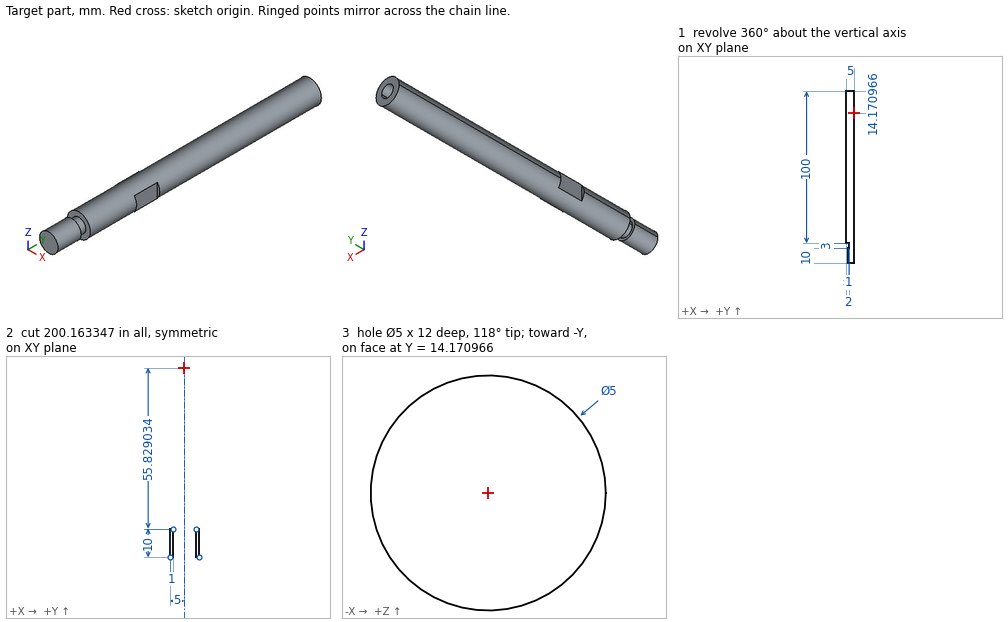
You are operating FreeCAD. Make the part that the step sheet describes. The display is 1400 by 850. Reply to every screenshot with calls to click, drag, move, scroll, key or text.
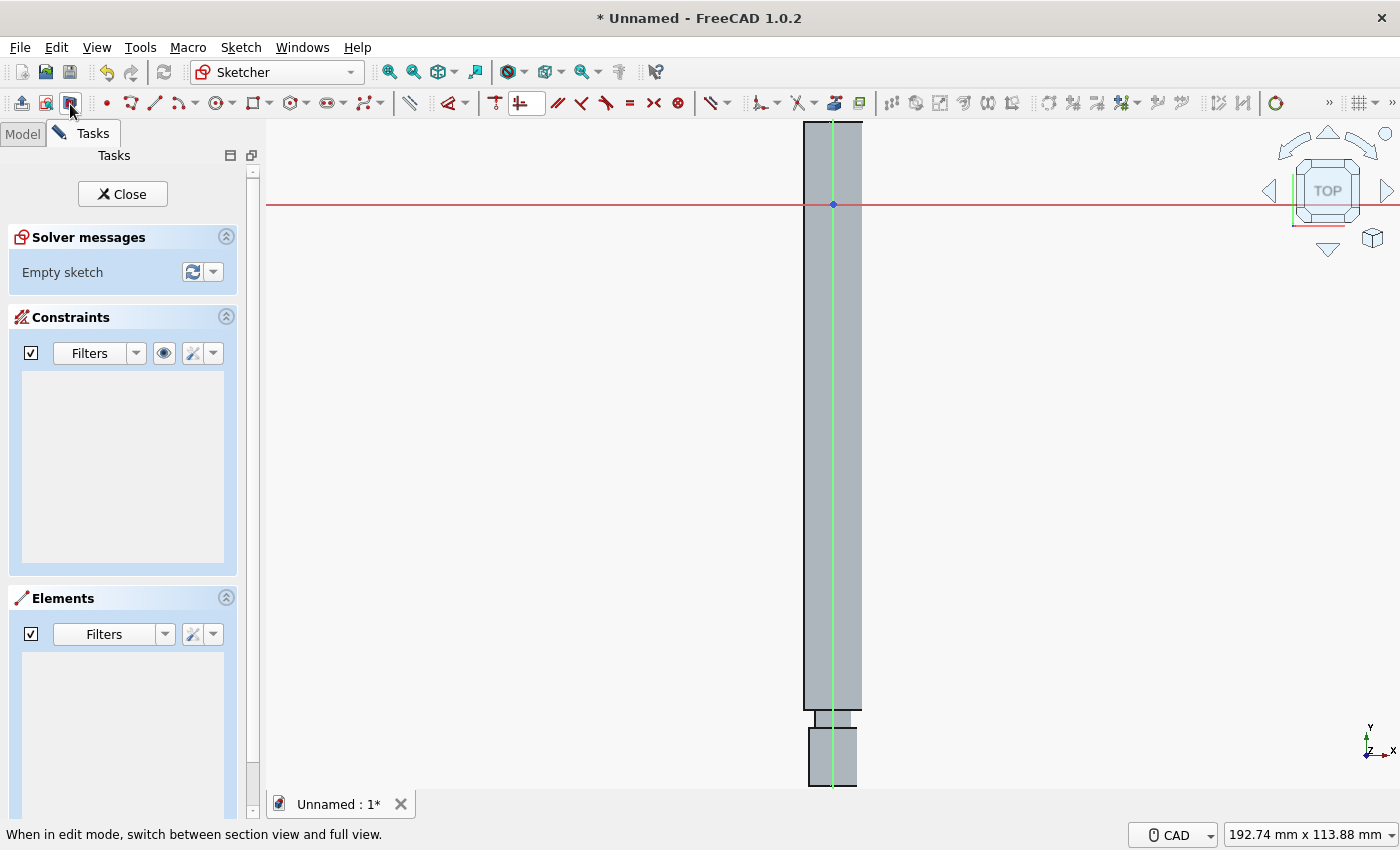
scroll(844, 580, up, 10)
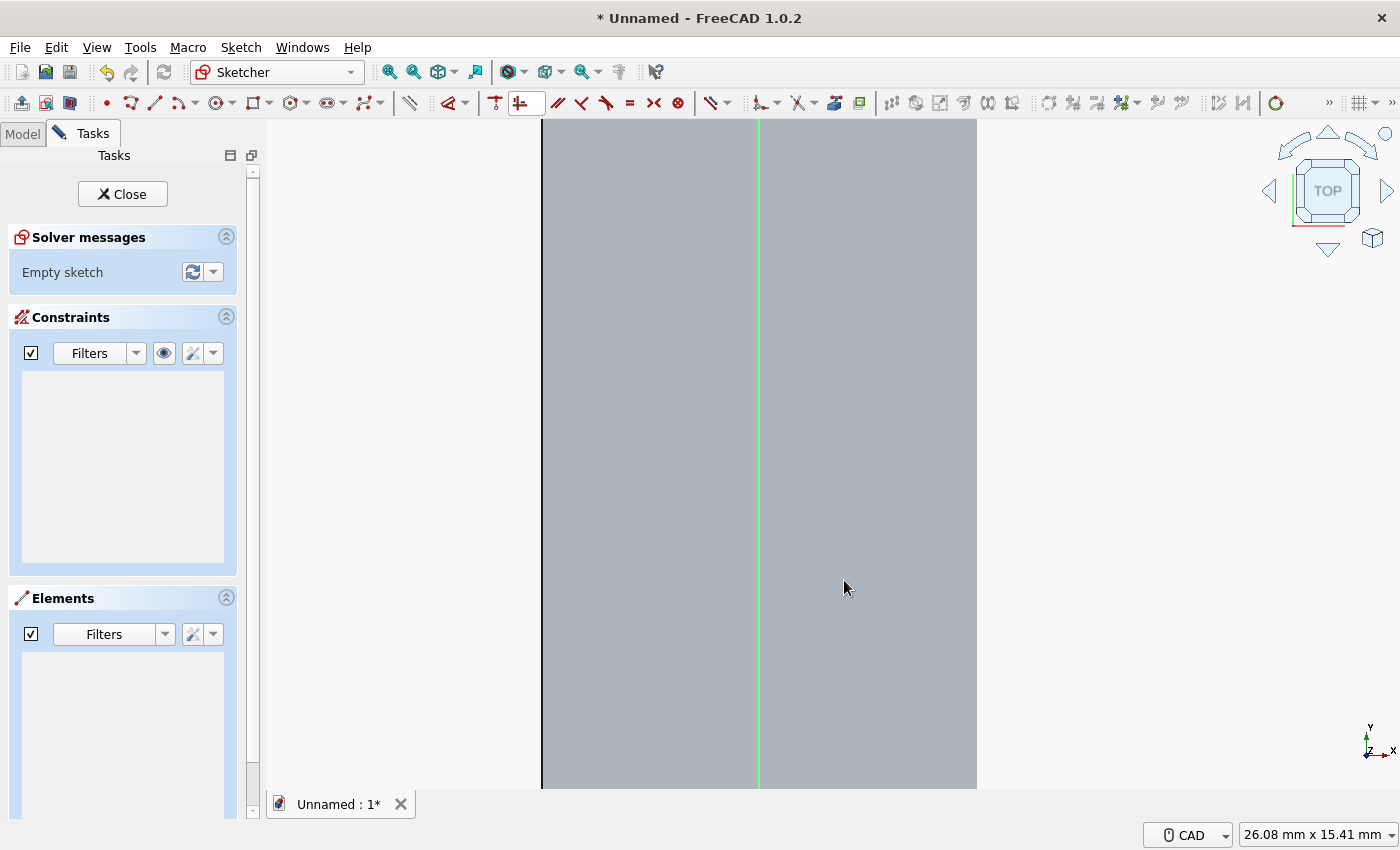
click(254, 104)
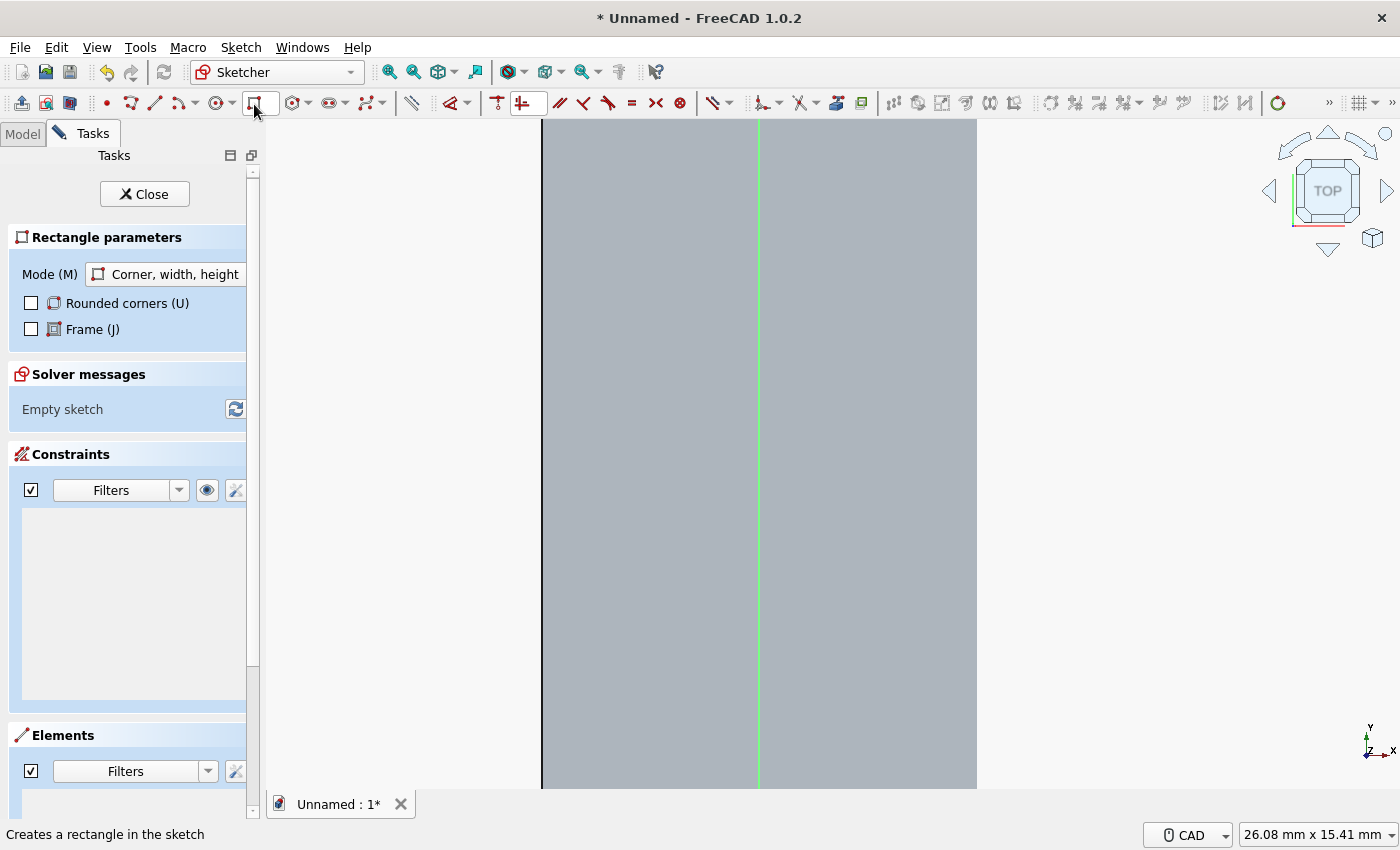
click(542, 231)
click(586, 666)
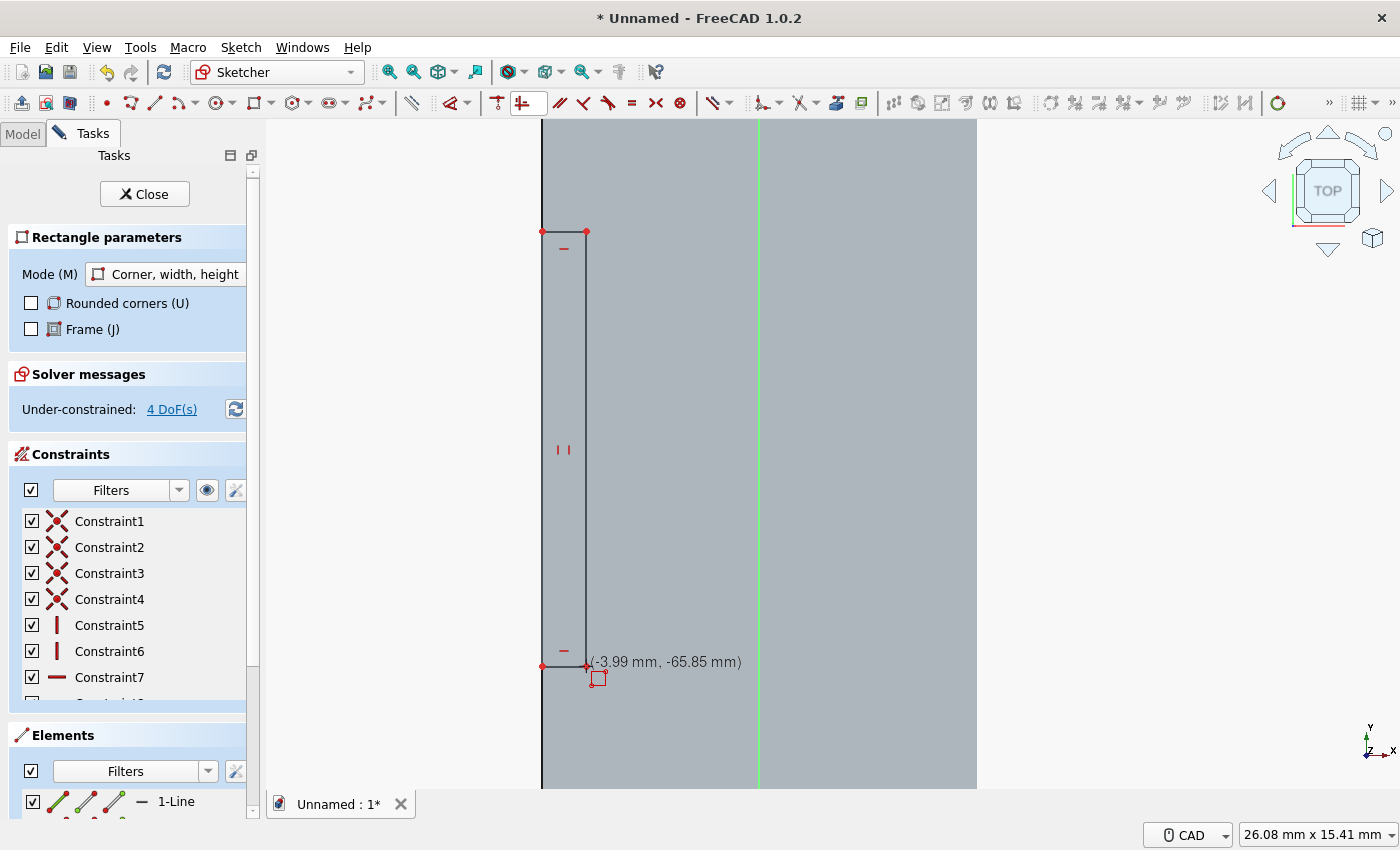
click(933, 231)
click(977, 666)
key(Escape)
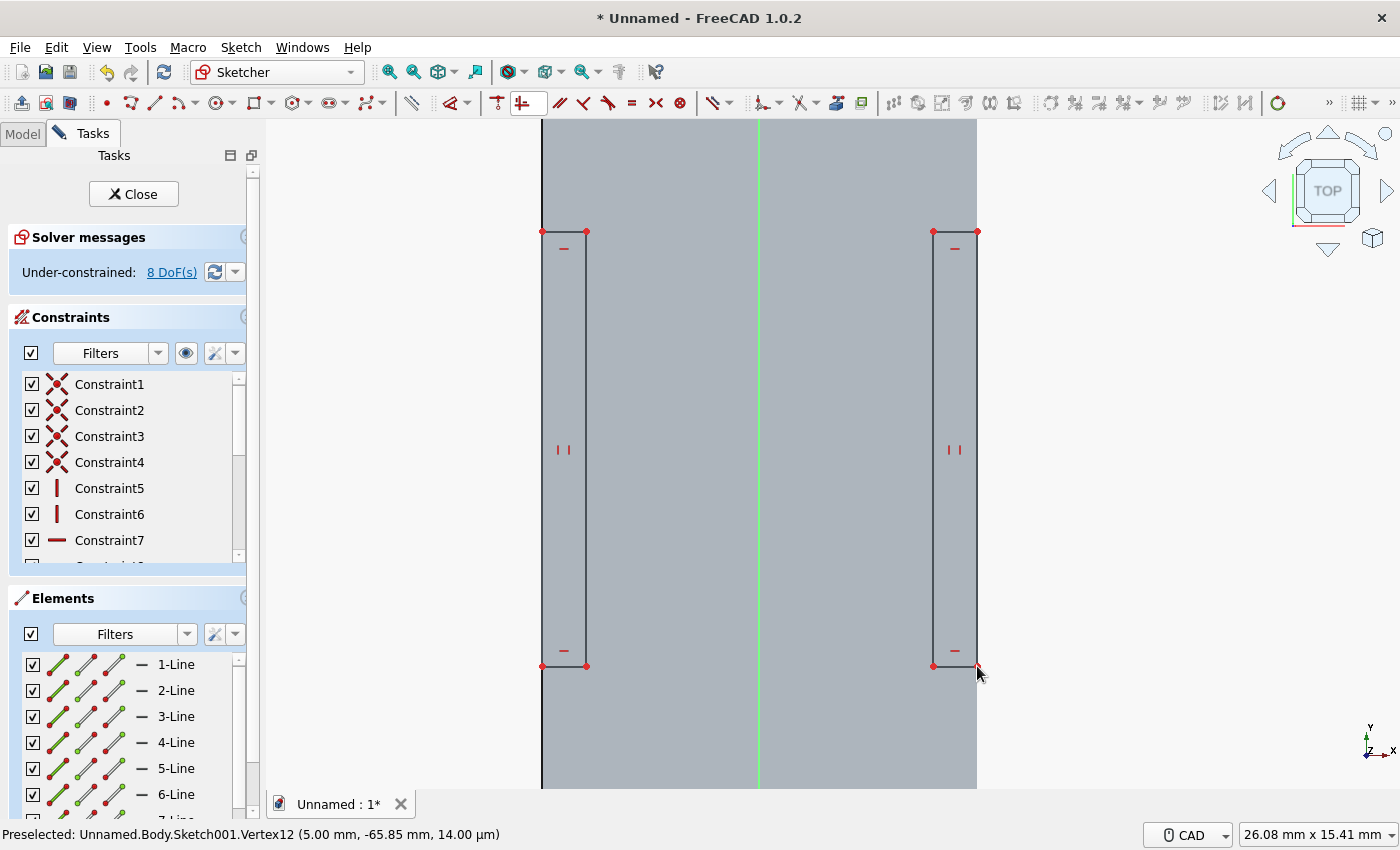
click(586, 232)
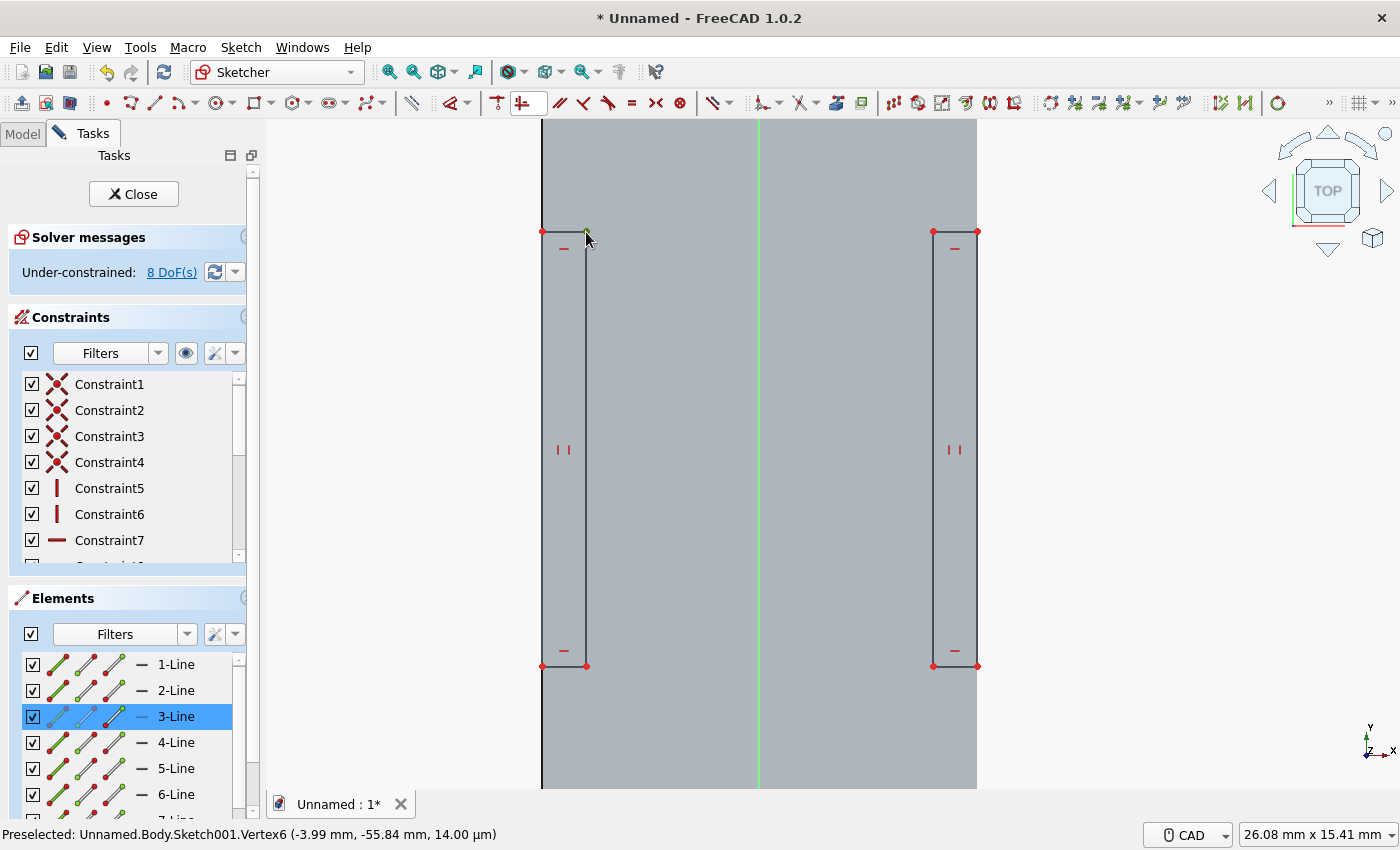
click(933, 232)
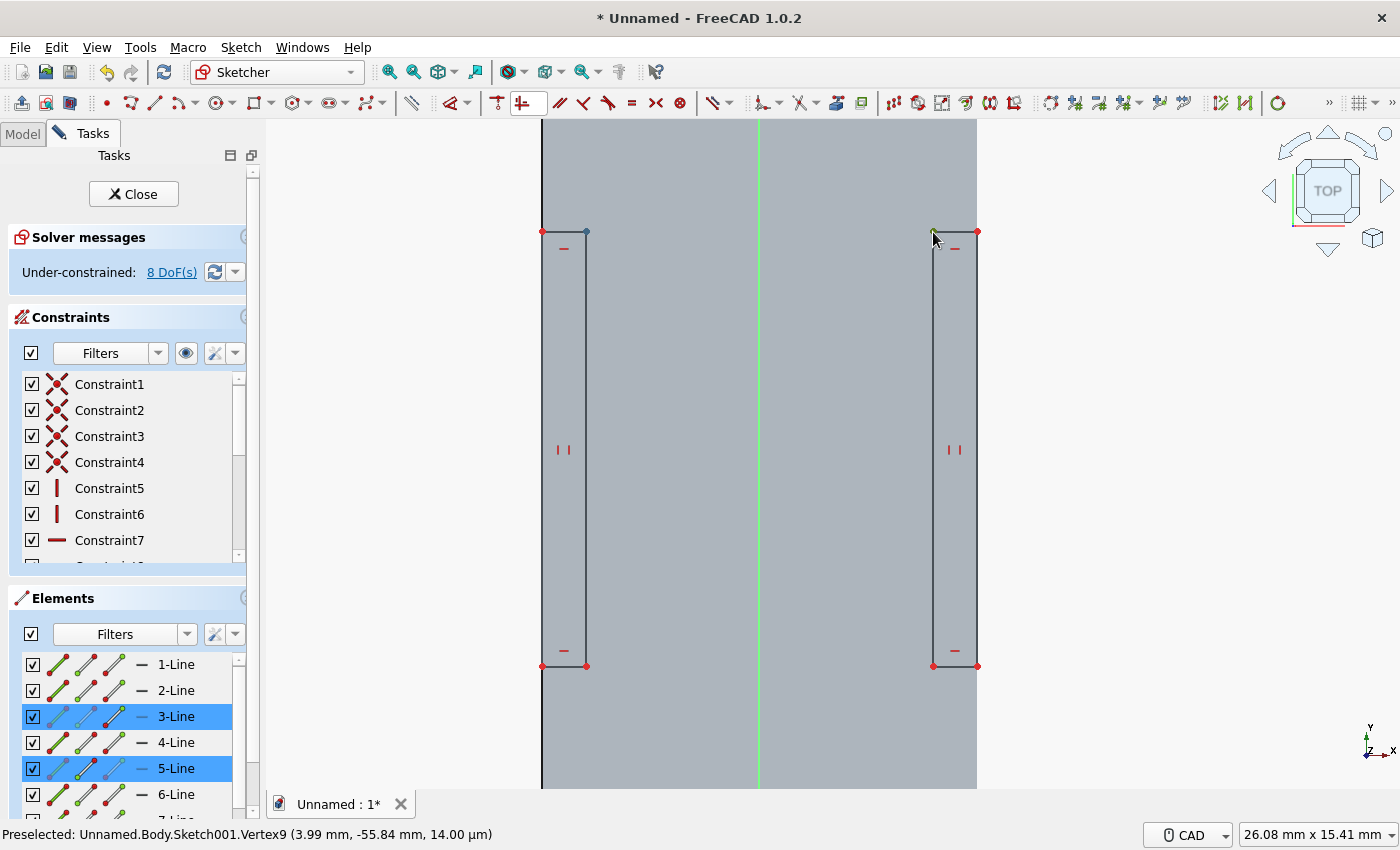
click(759, 717)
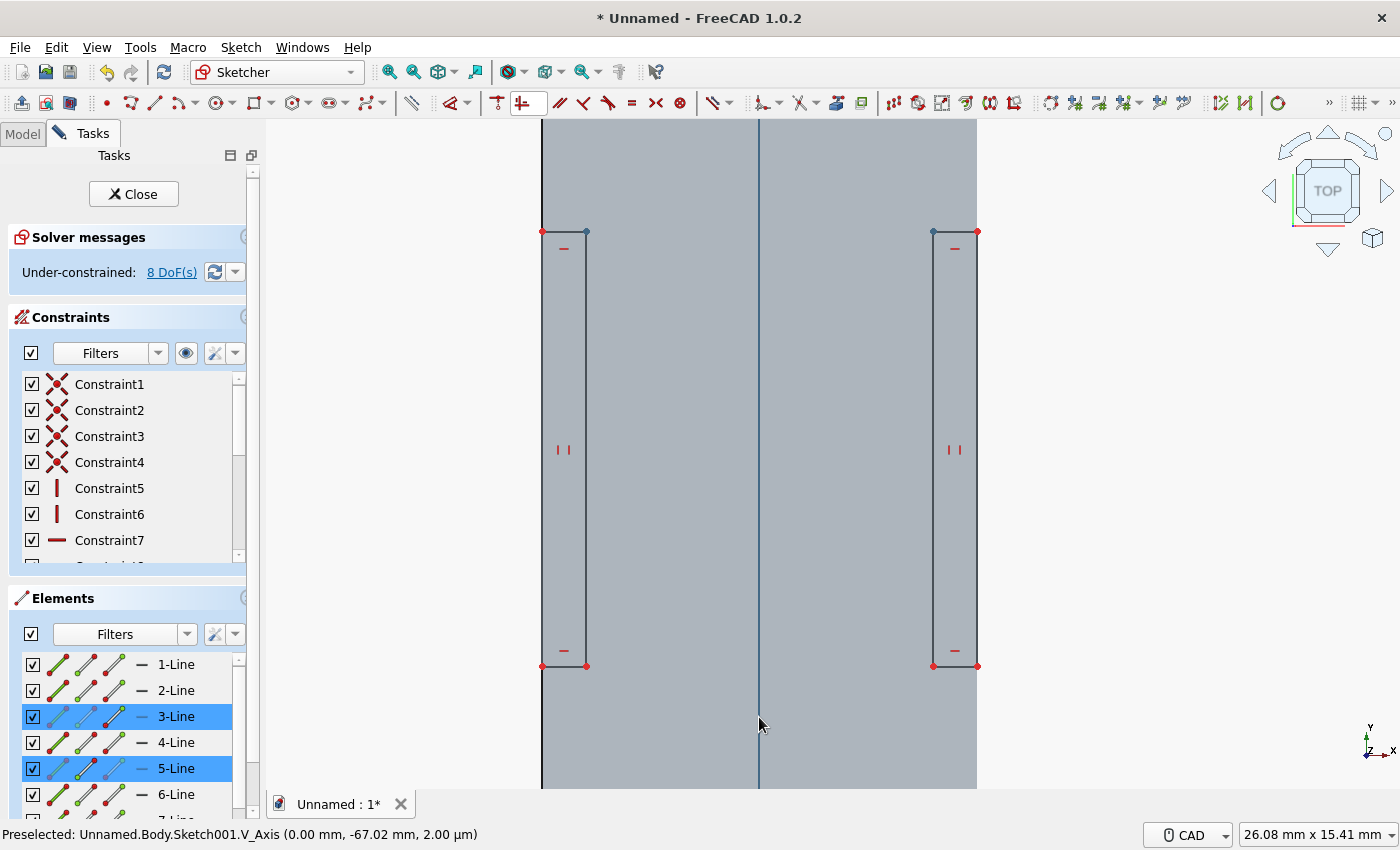
click(656, 104)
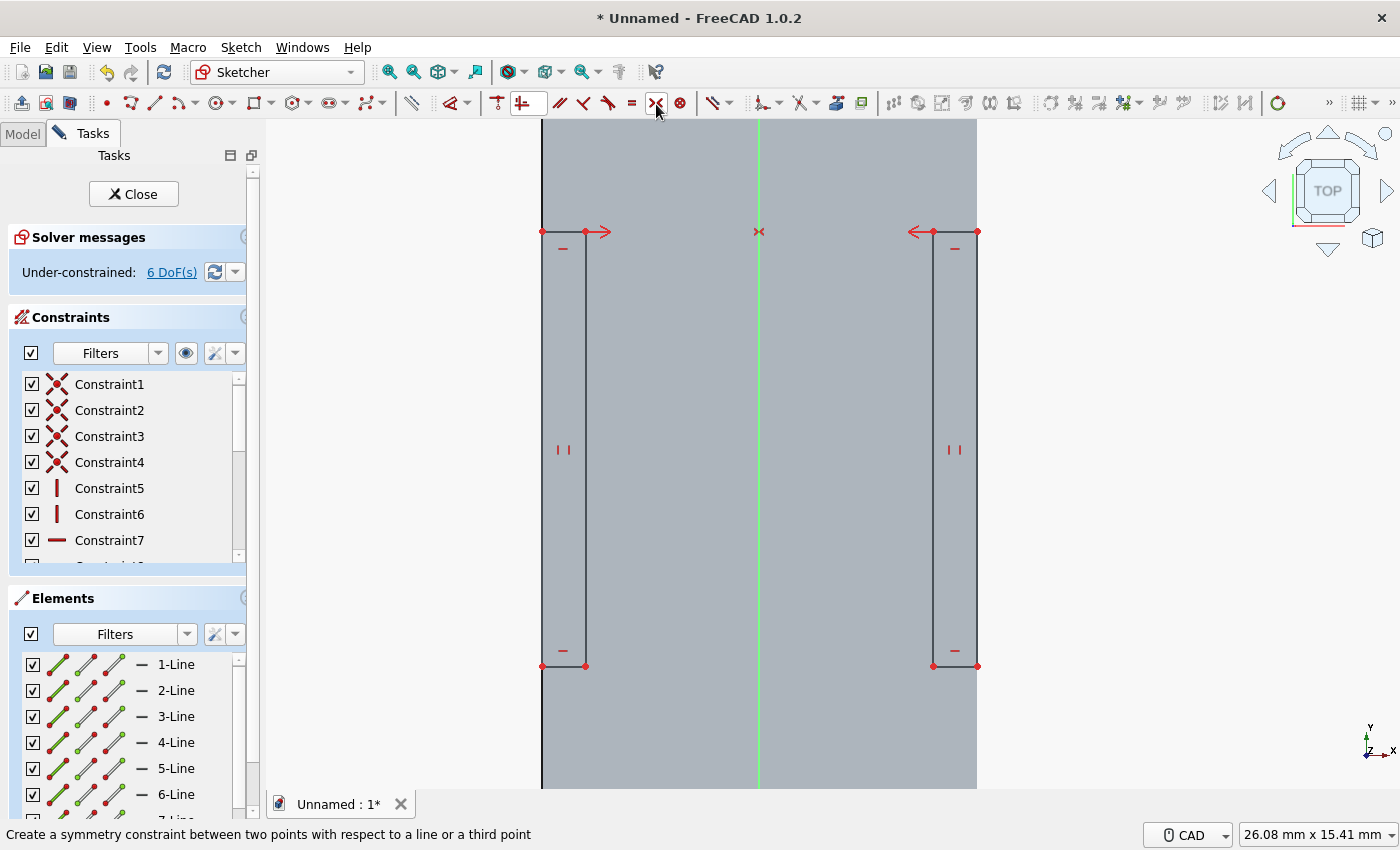
click(542, 667)